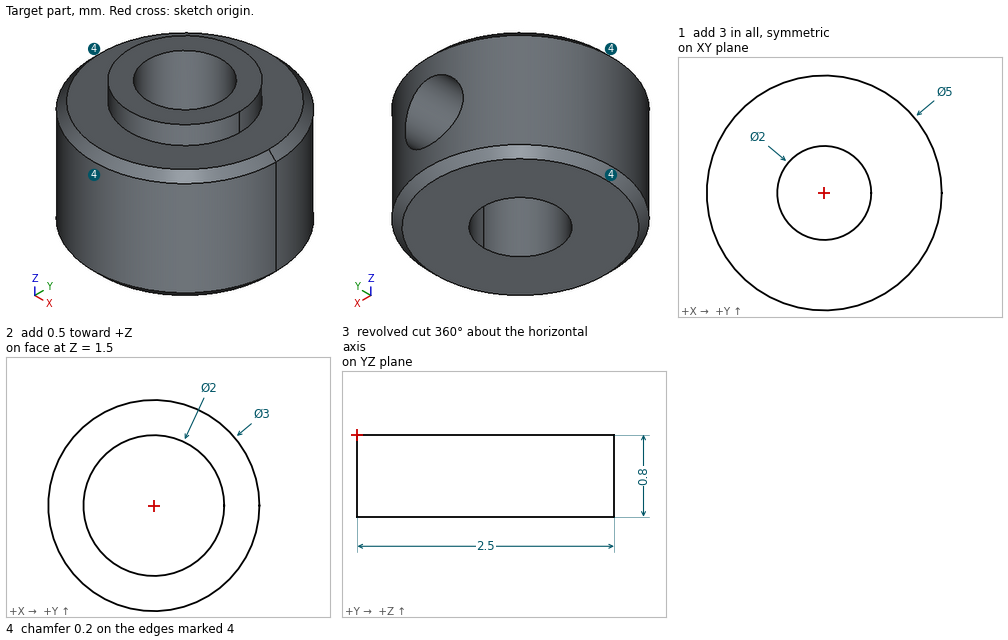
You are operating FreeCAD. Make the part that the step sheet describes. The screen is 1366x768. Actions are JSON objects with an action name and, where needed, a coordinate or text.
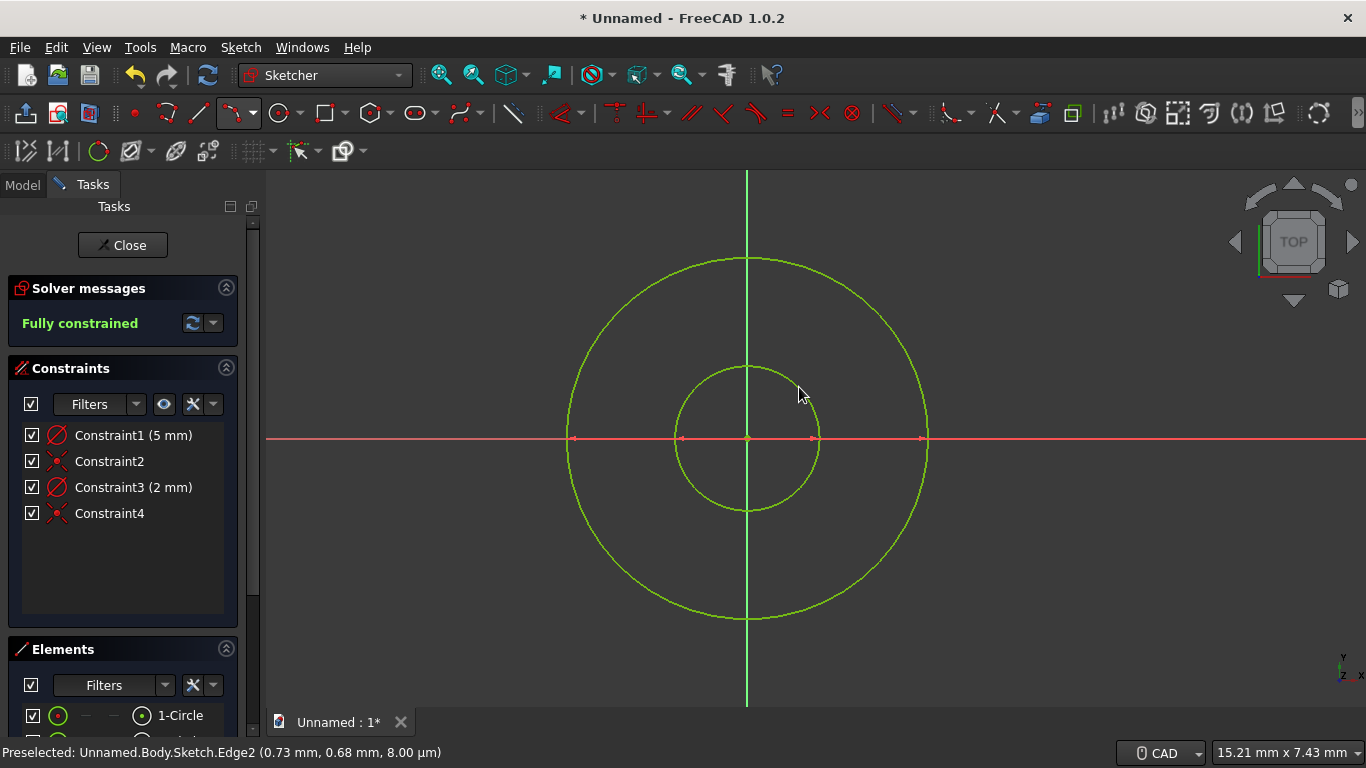
{"action": "left_click", "coordinate": [123, 245]}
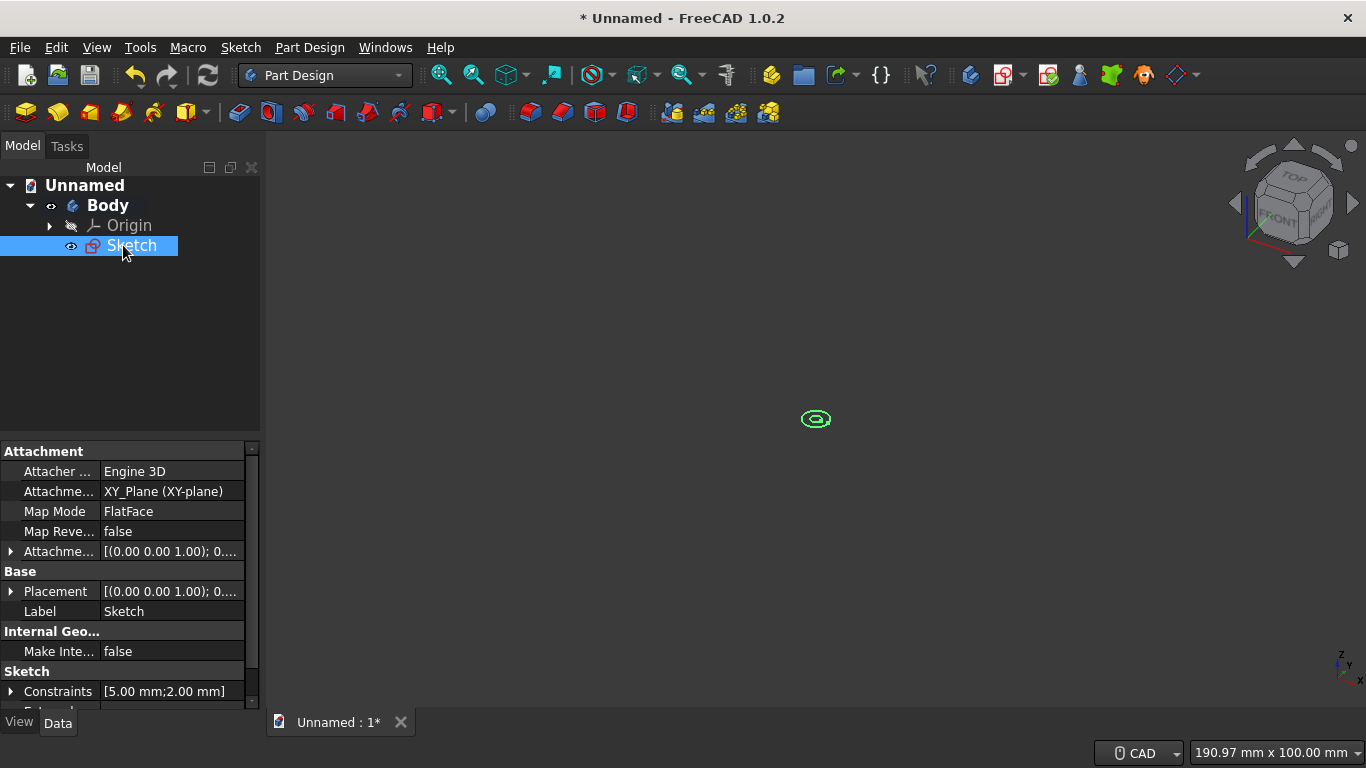
{"action": "left_click", "coordinate": [26, 112]}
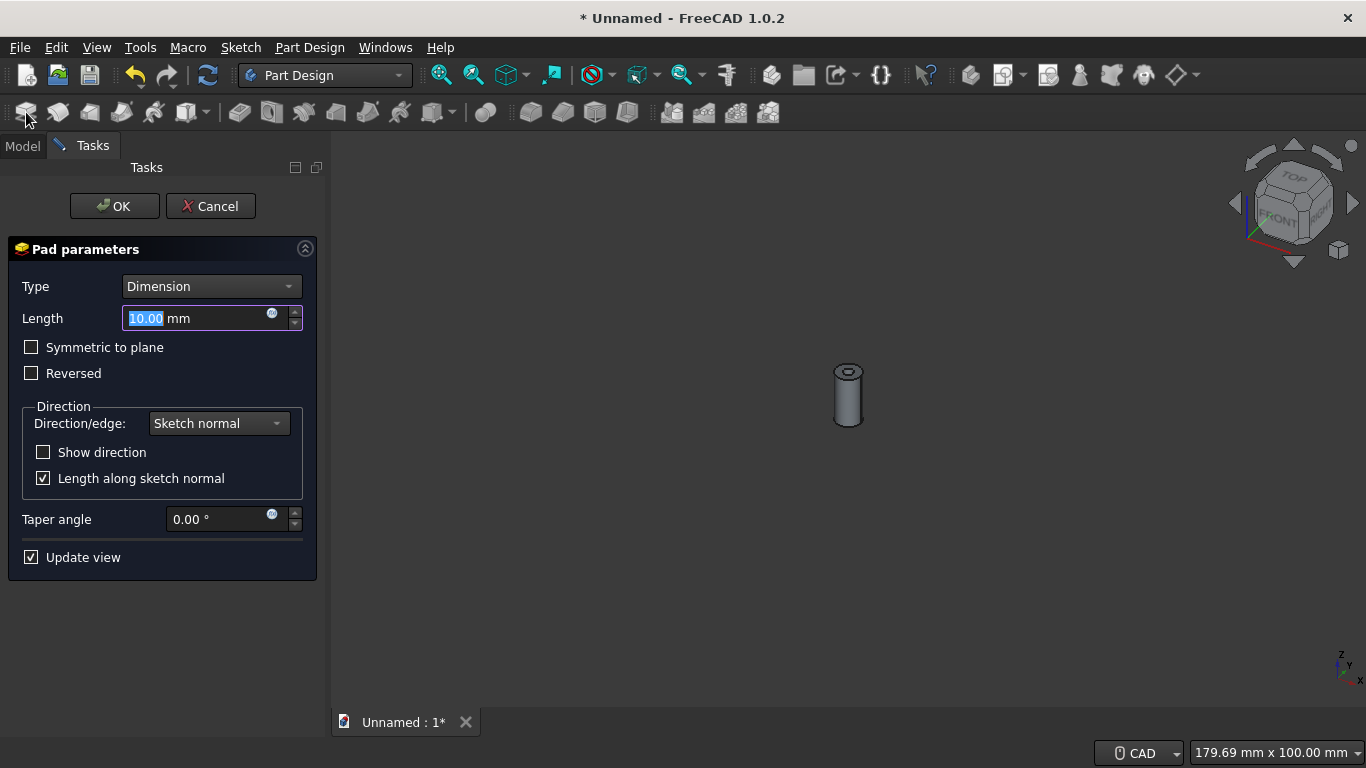
{"action": "type", "text": "3"}
{"action": "key", "text": "Tab"}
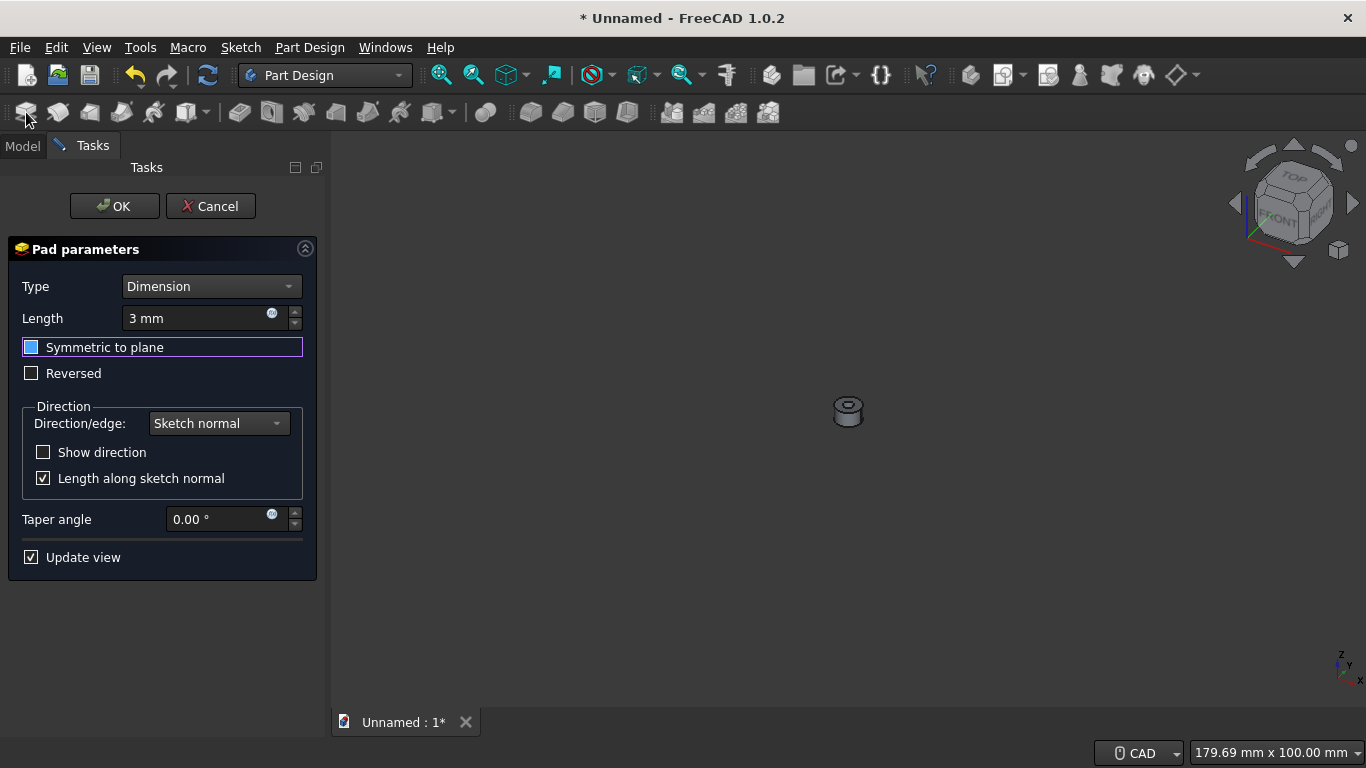
{"action": "left_click", "coordinate": [30, 347]}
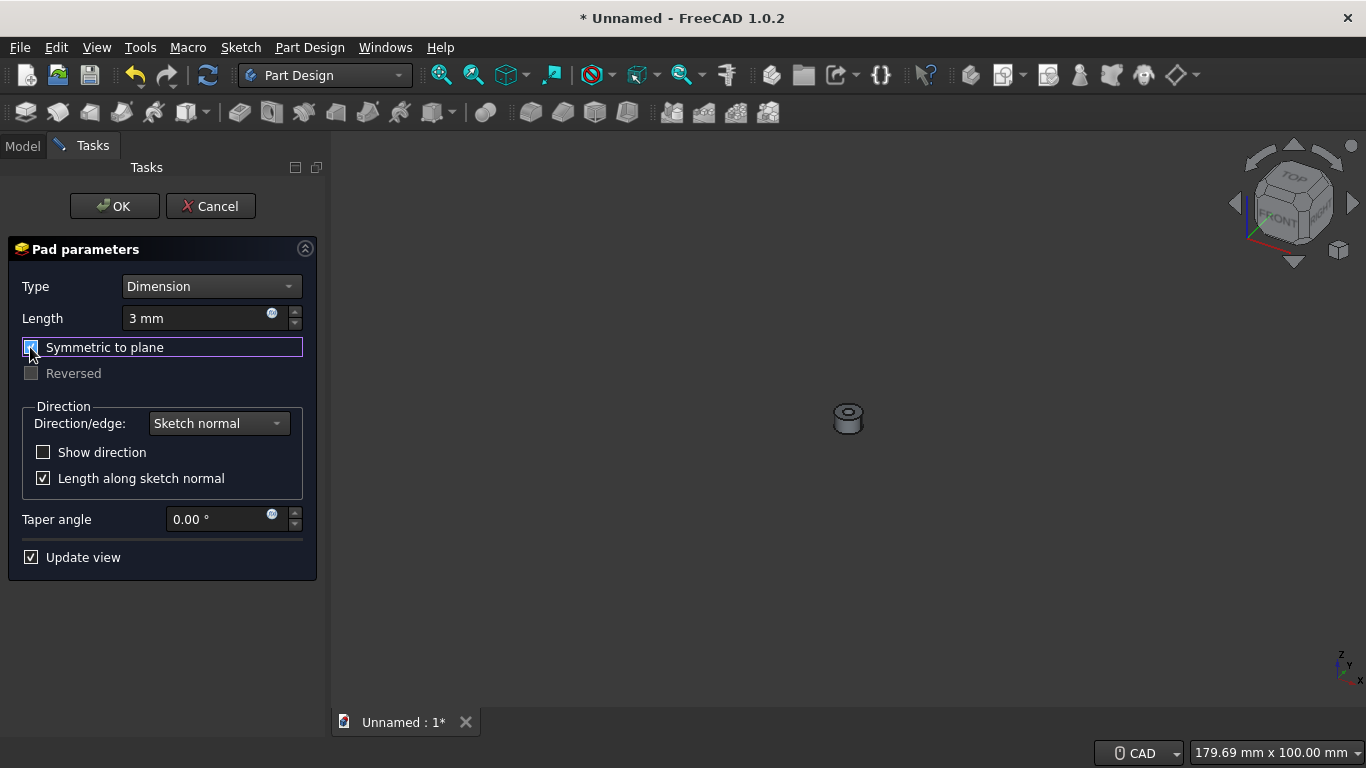
{"action": "left_click", "coordinate": [115, 206]}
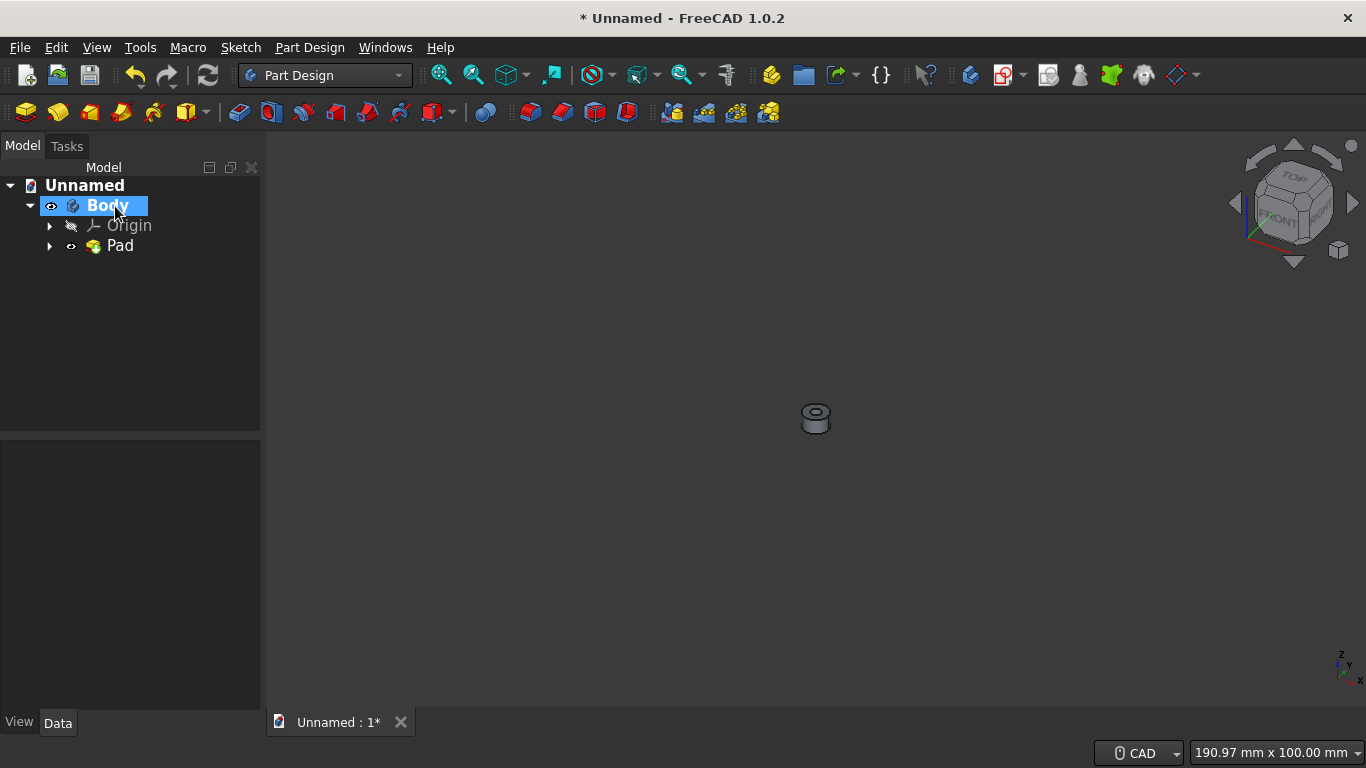
{"action": "left_click", "coordinate": [442, 76]}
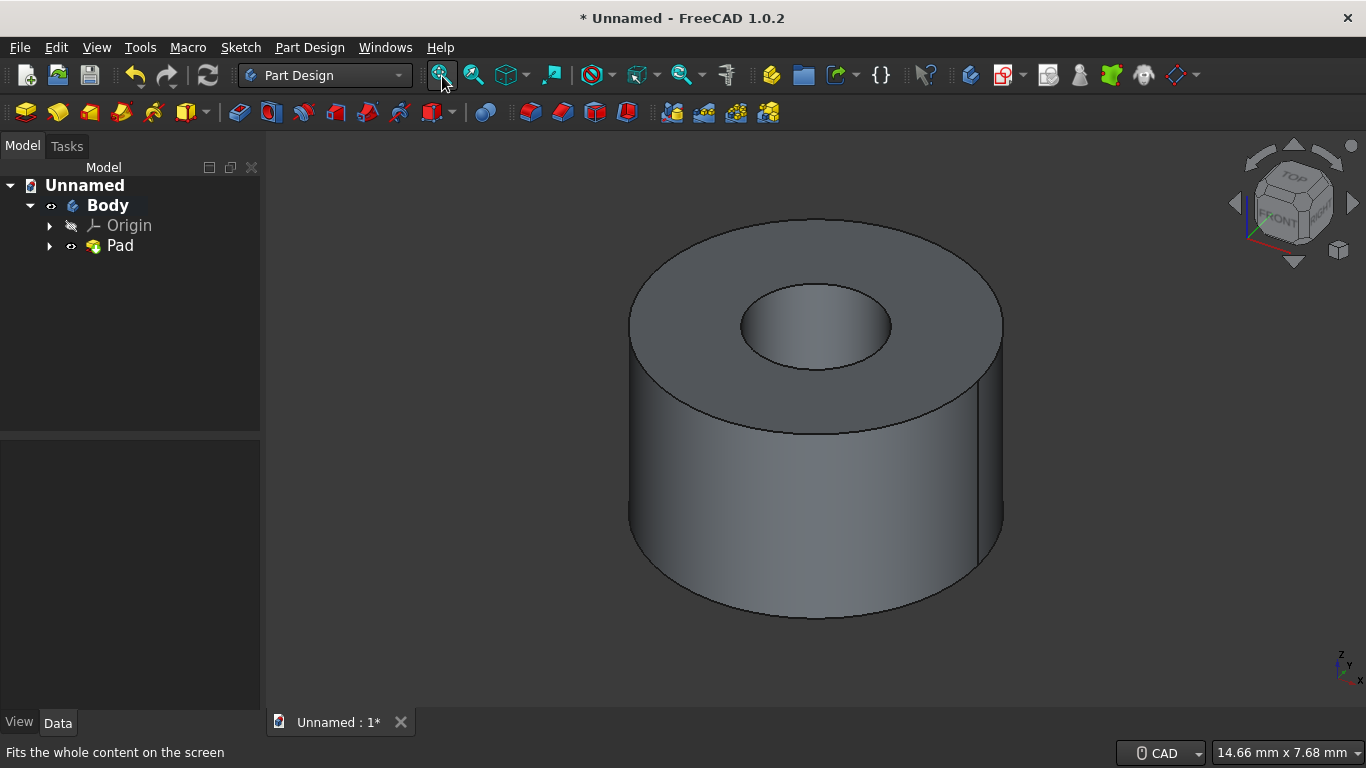
{"action": "left_click", "coordinate": [750, 268]}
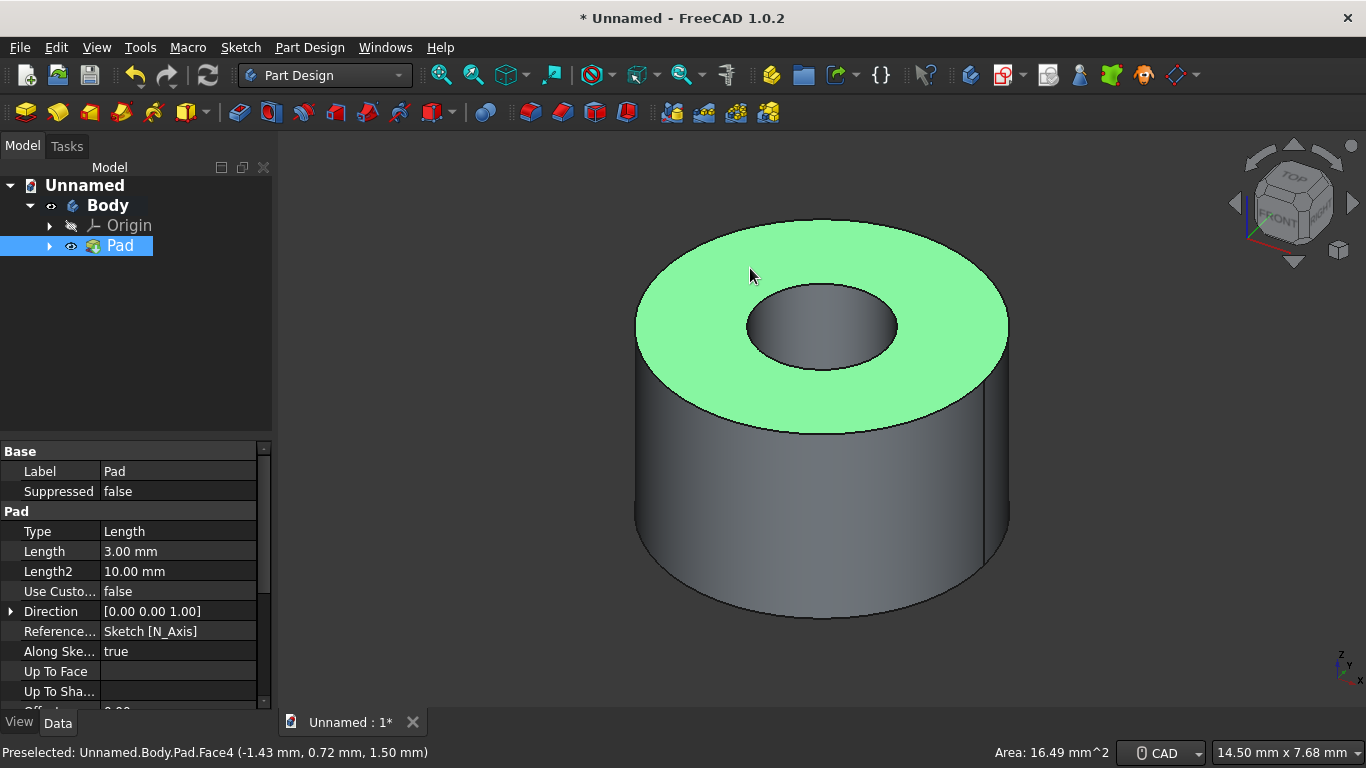
{"action": "left_click", "coordinate": [1004, 76]}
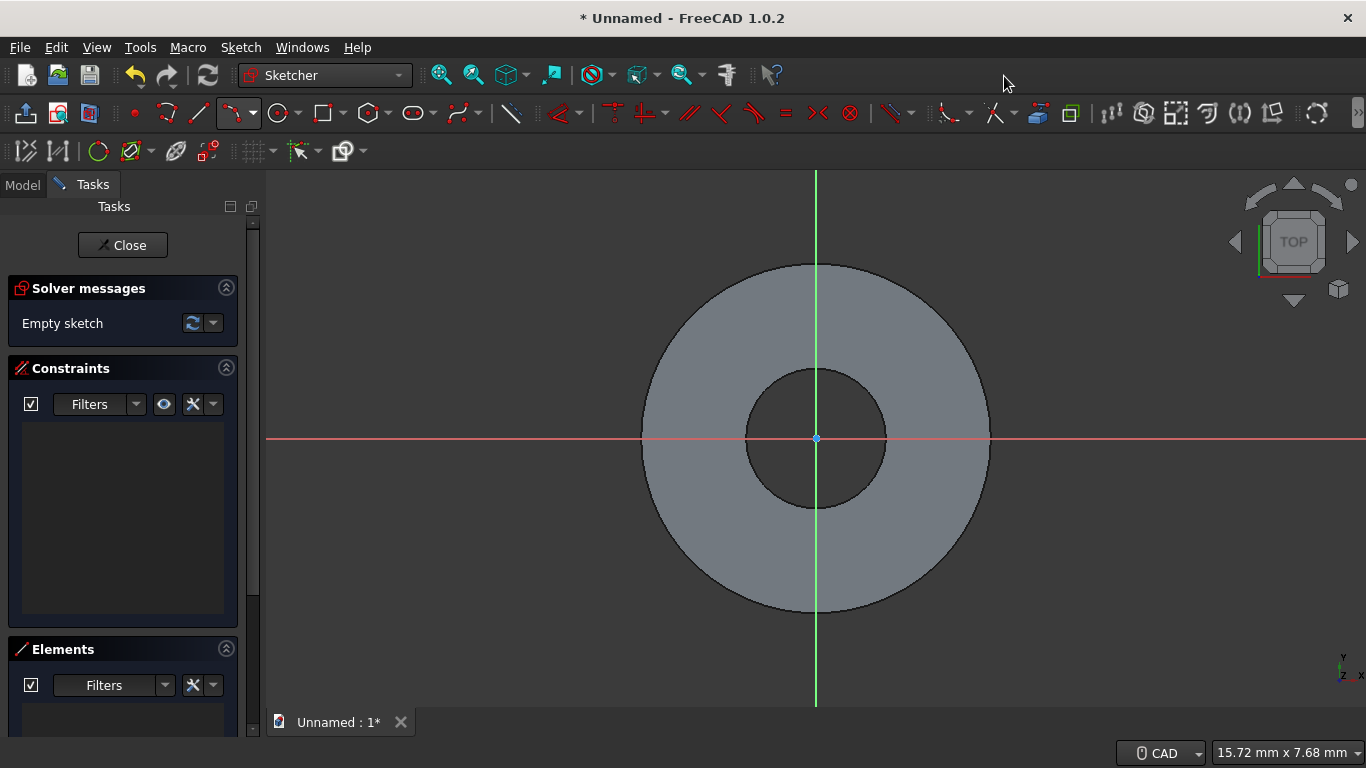
{"action": "scroll", "coordinate": [955, 439], "scroll_direction": "up", "scroll_amount": 2}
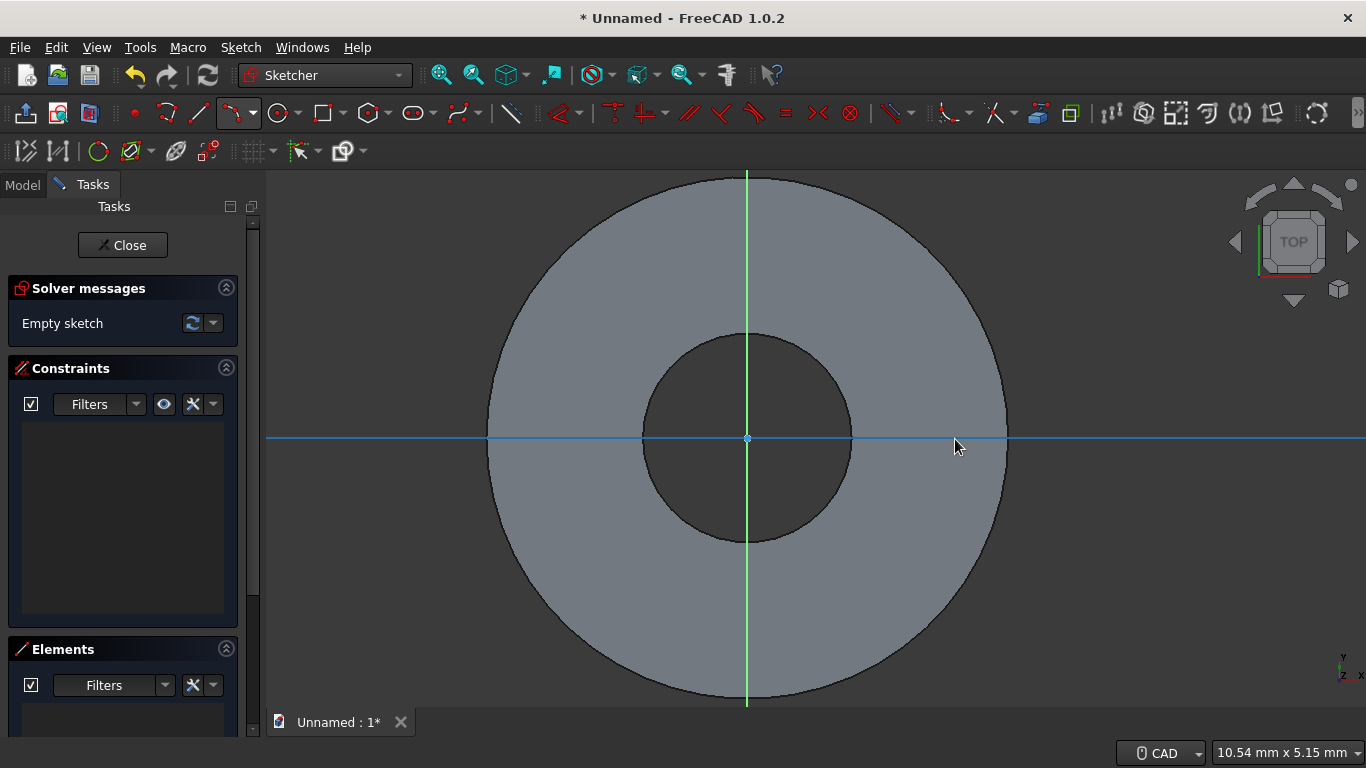
{"action": "left_click", "coordinate": [278, 114]}